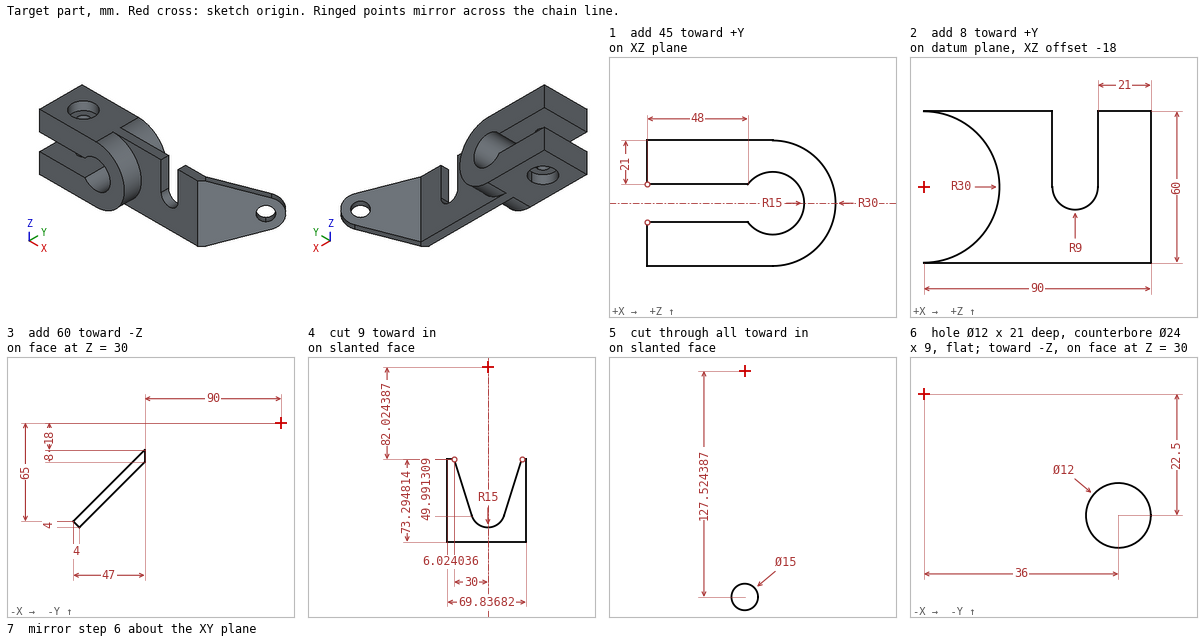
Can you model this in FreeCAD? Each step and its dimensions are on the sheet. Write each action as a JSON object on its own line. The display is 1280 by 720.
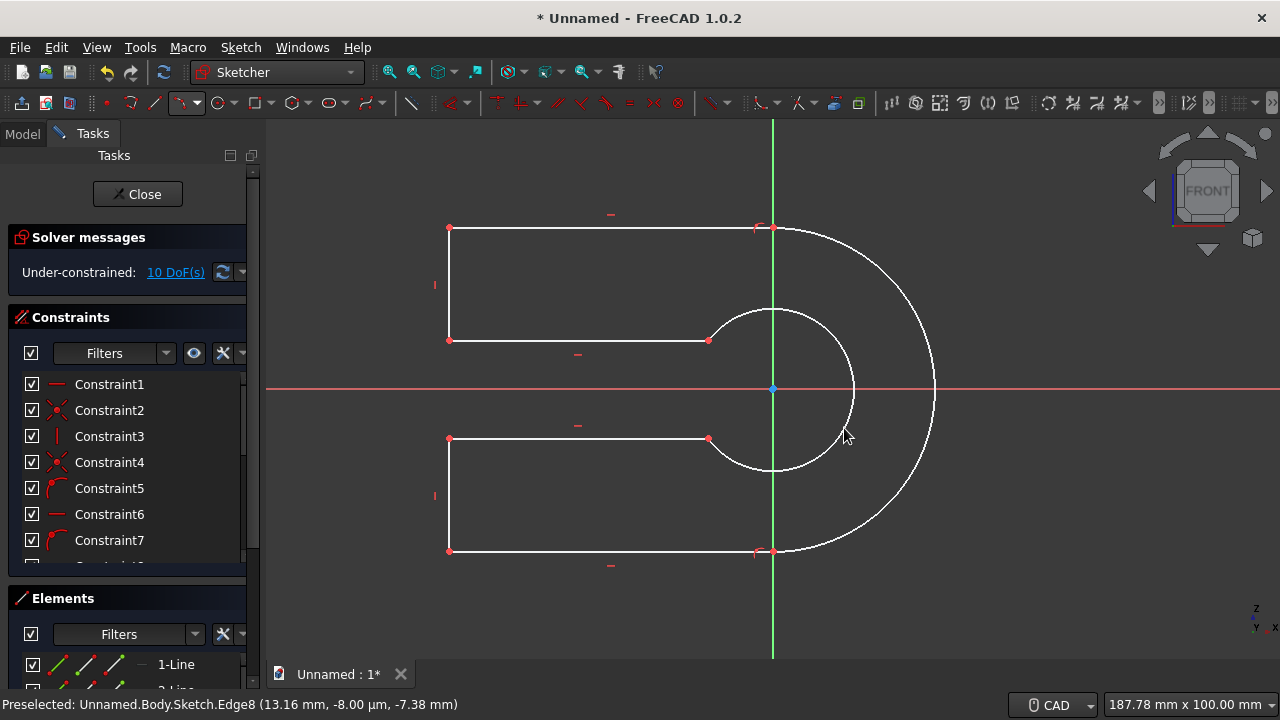
{"action": "left_click", "coordinate": [904, 485]}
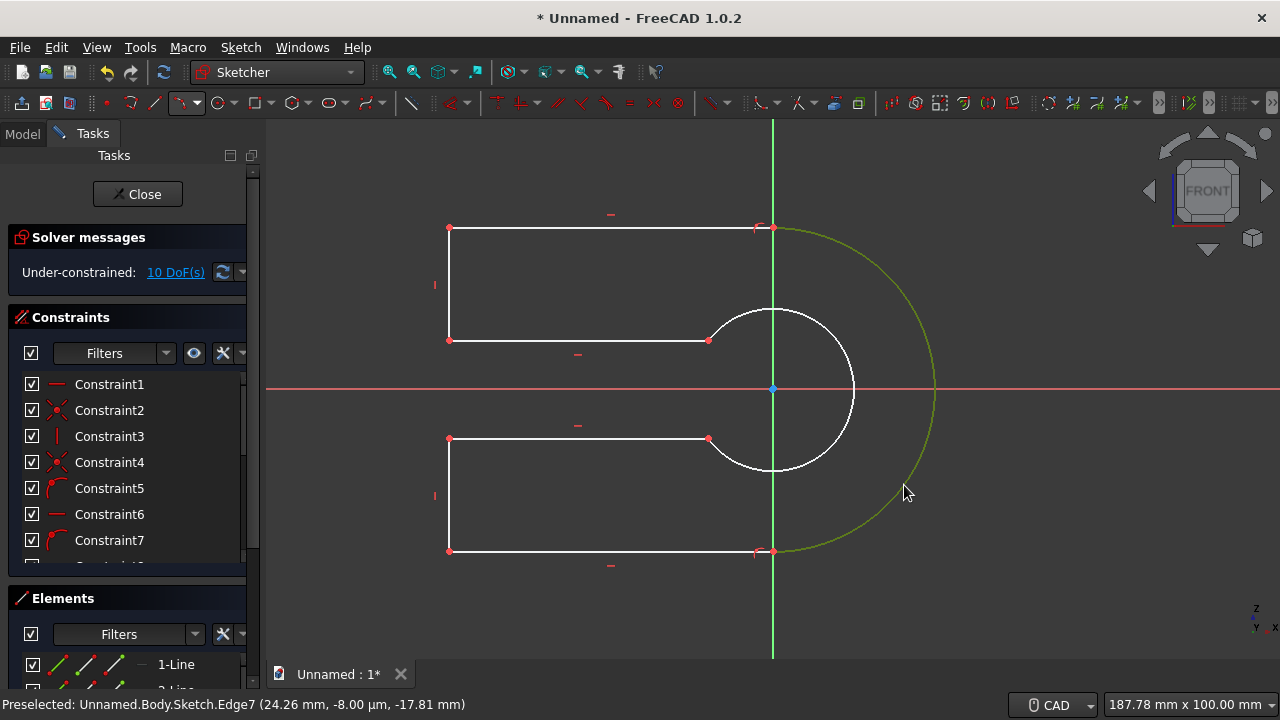
{"action": "left_click", "coordinate": [817, 458]}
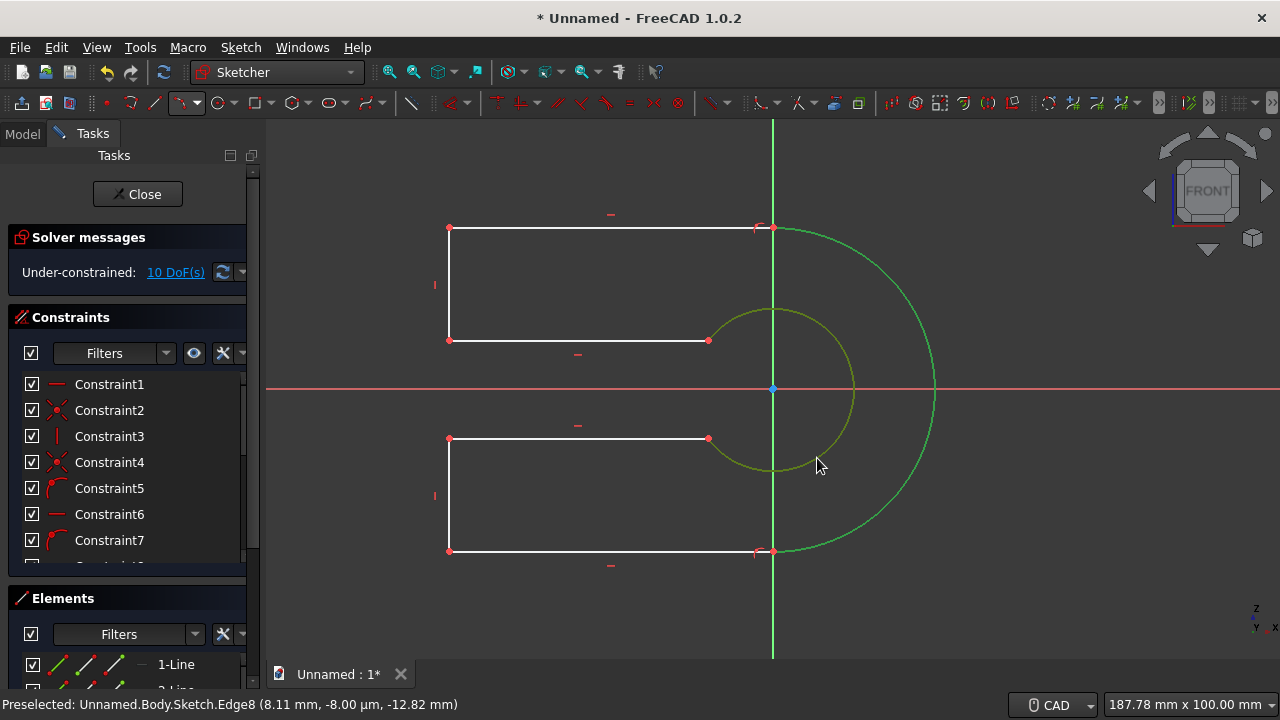
{"action": "left_click", "coordinate": [498, 104]}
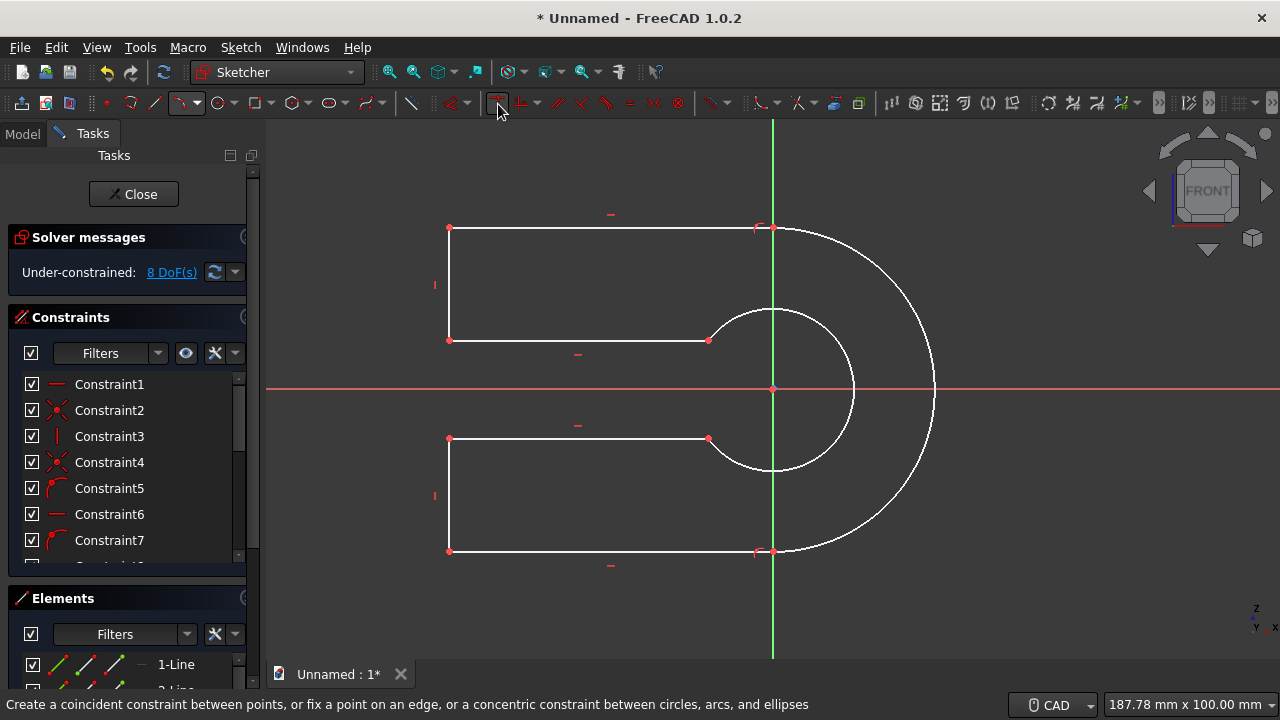
{"action": "left_click_drag", "start_coordinate": [763, 379], "coordinate": [783, 400]}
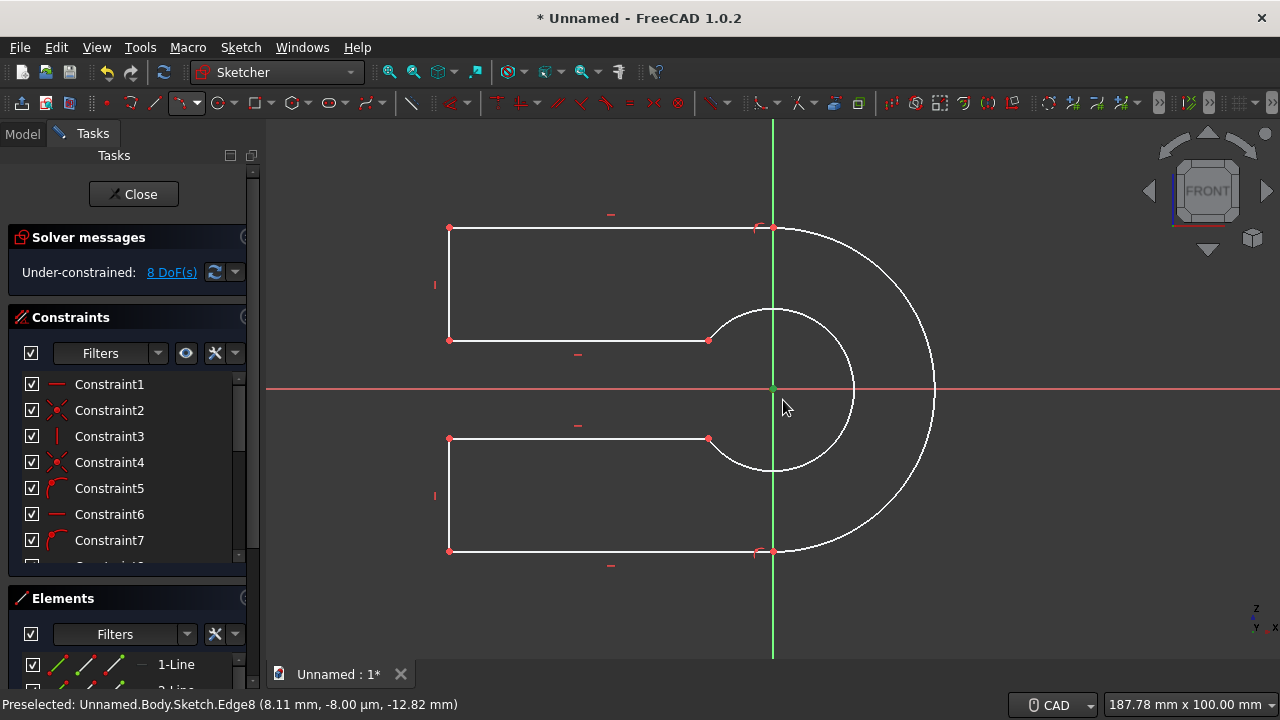
{"action": "left_click", "coordinate": [498, 104]}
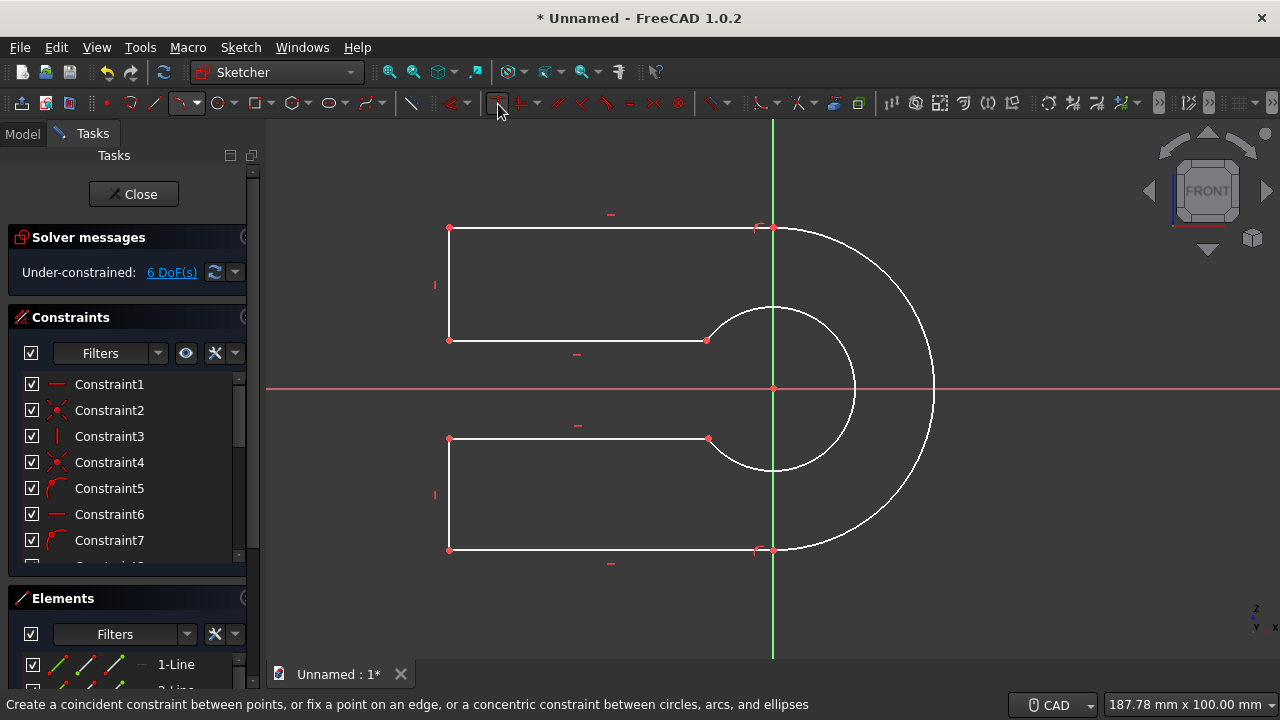
{"action": "left_click", "coordinate": [449, 341]}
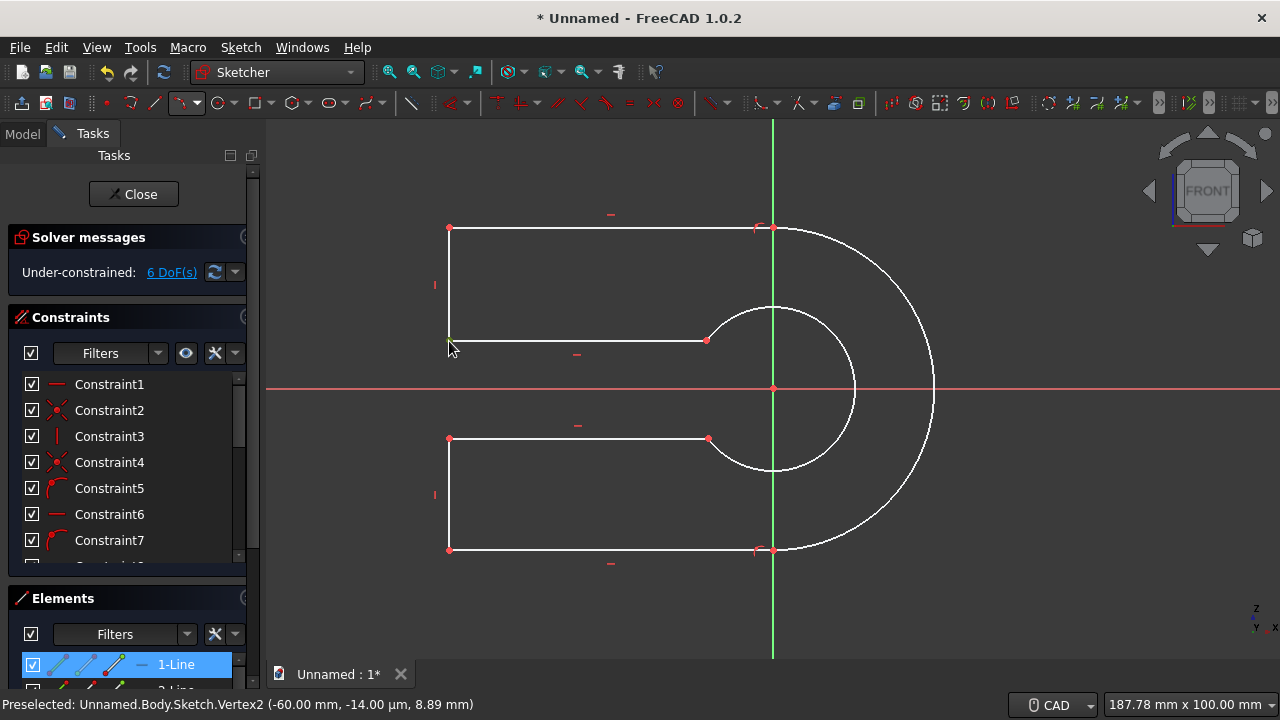
{"action": "left_click", "coordinate": [449, 439]}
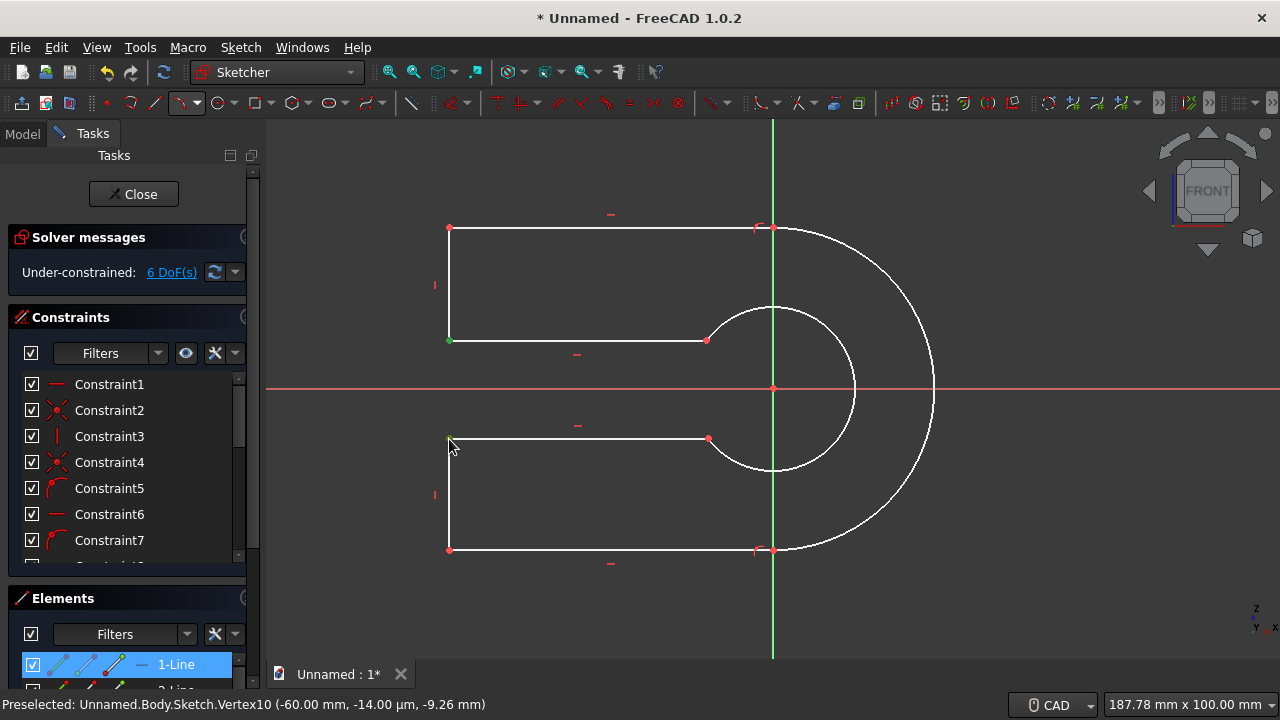
{"action": "left_click", "coordinate": [353, 389]}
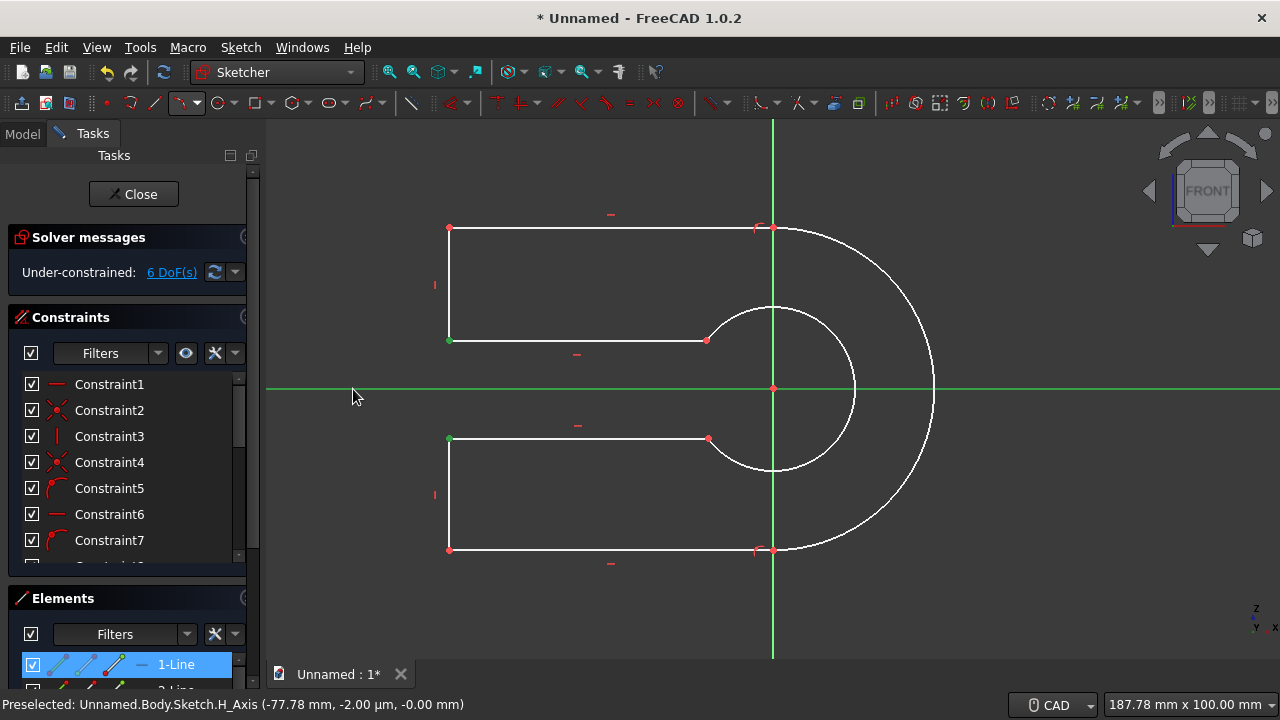
{"action": "key", "text": "s"}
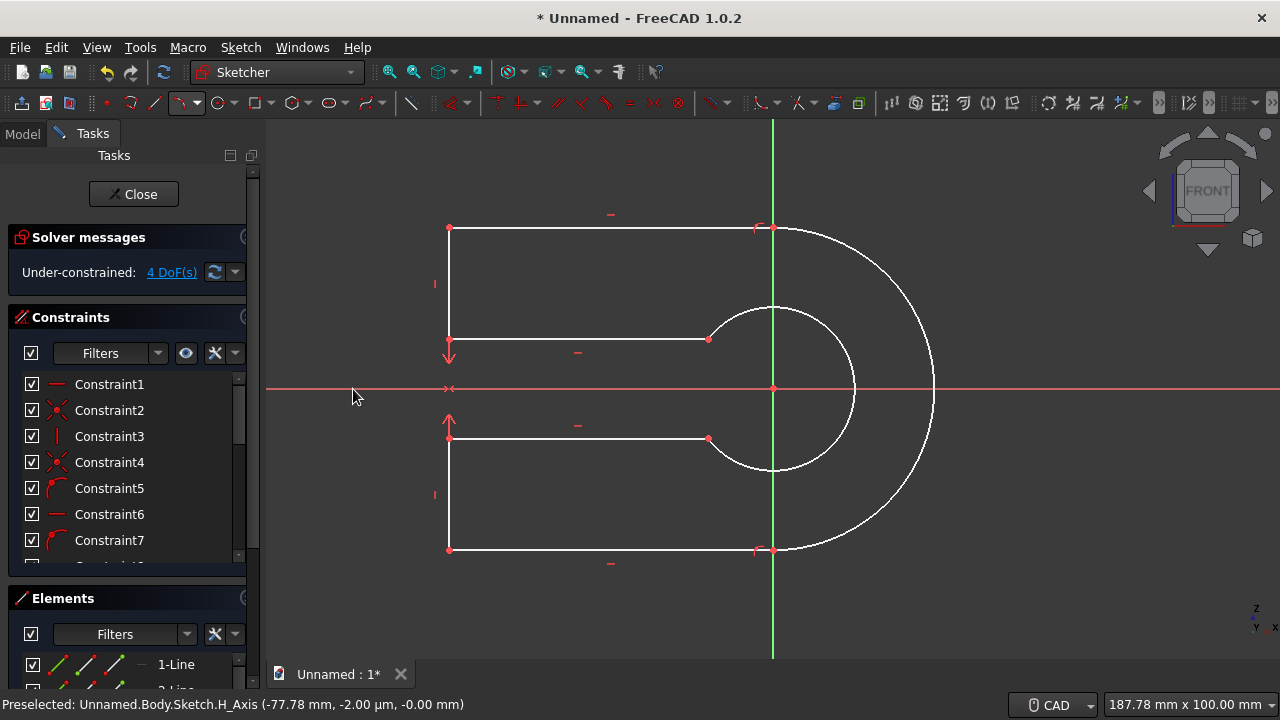
{"action": "left_click", "coordinate": [450, 104]}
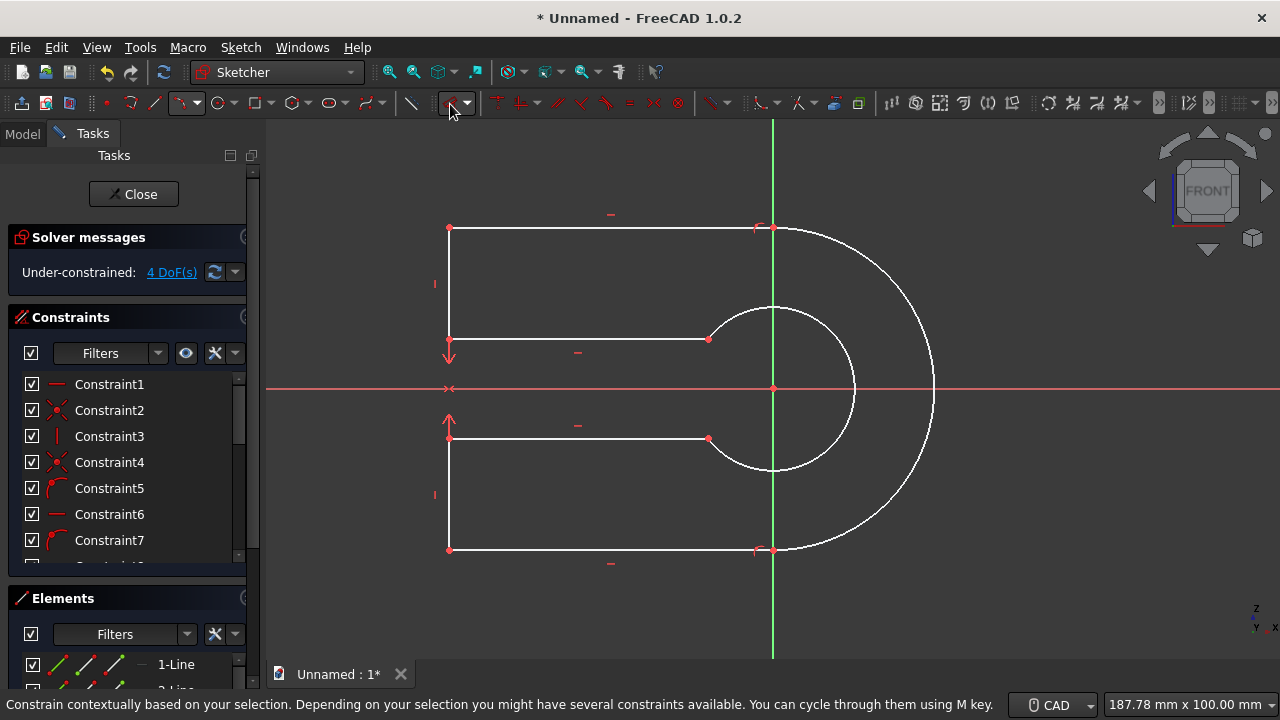
{"action": "left_click", "coordinate": [903, 484]}
{"action": "left_click", "coordinate": [929, 503]}